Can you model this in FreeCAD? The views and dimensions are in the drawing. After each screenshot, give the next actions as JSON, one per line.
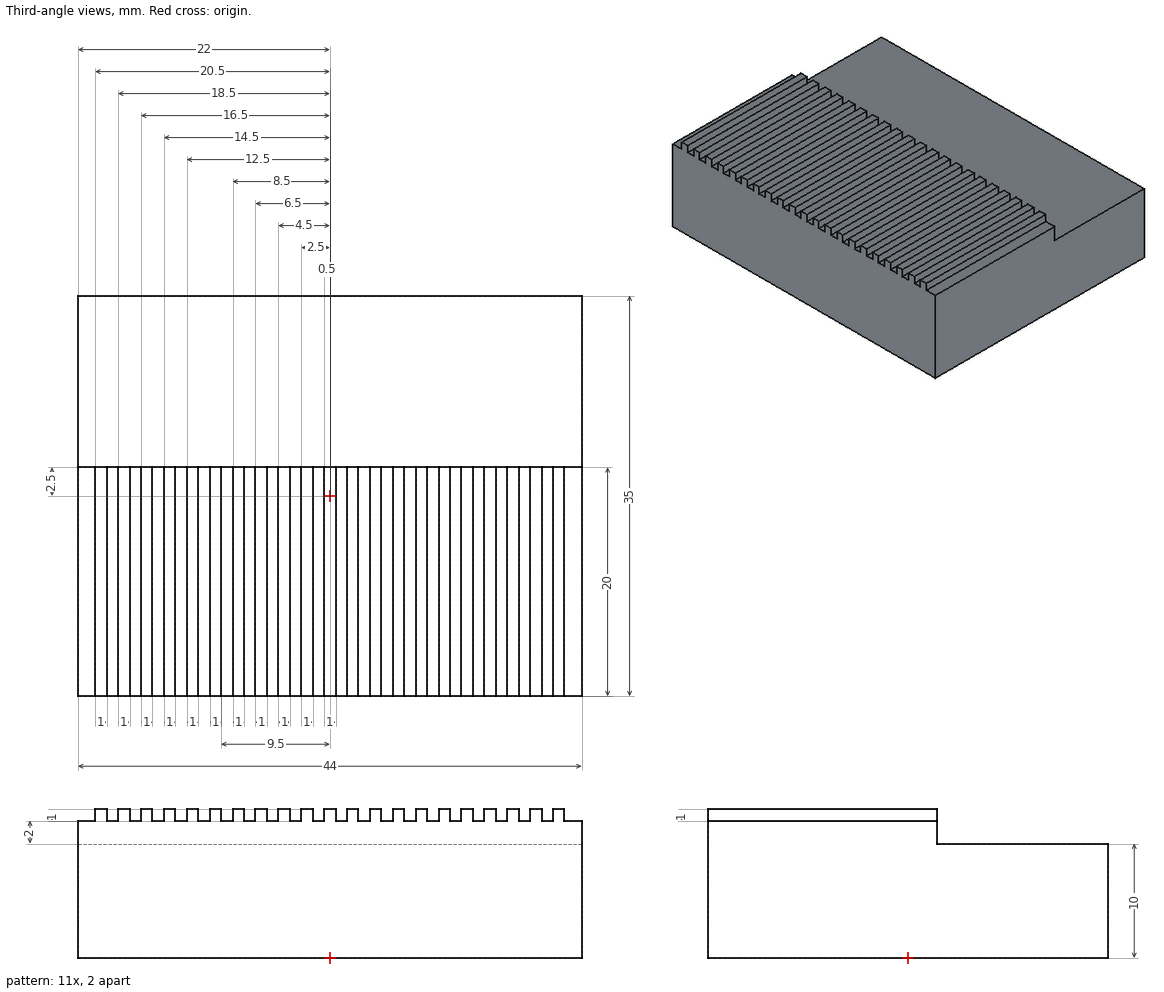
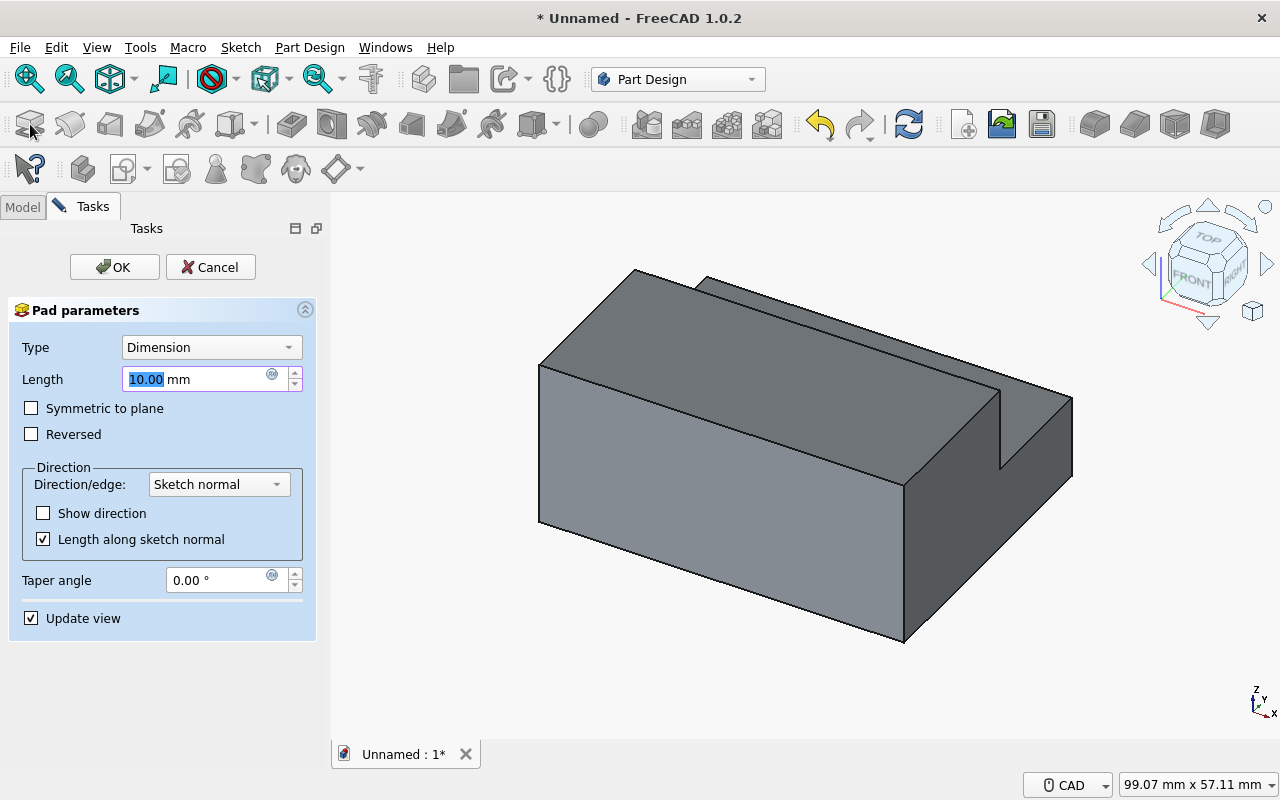
{"action": "type", "text": "2"}
{"action": "key", "text": "Tab"}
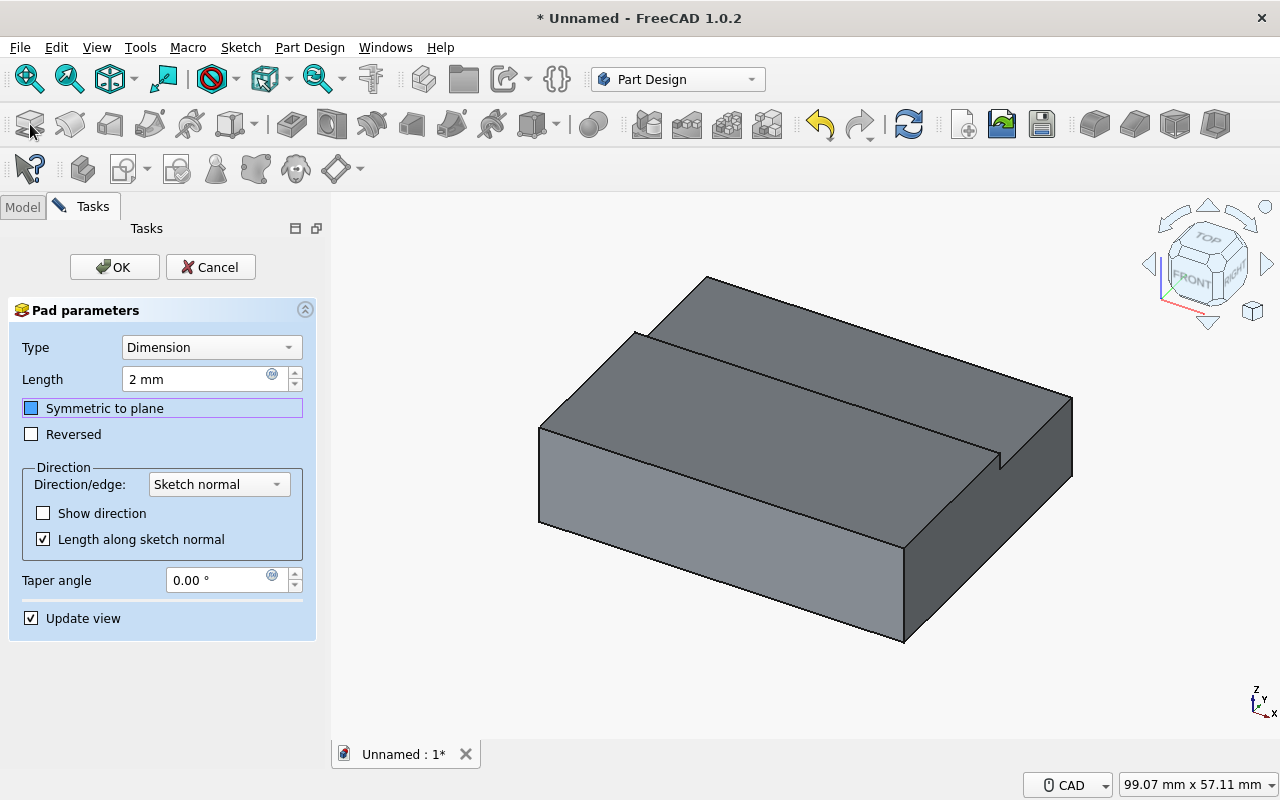
{"action": "left_click", "coordinate": [115, 267]}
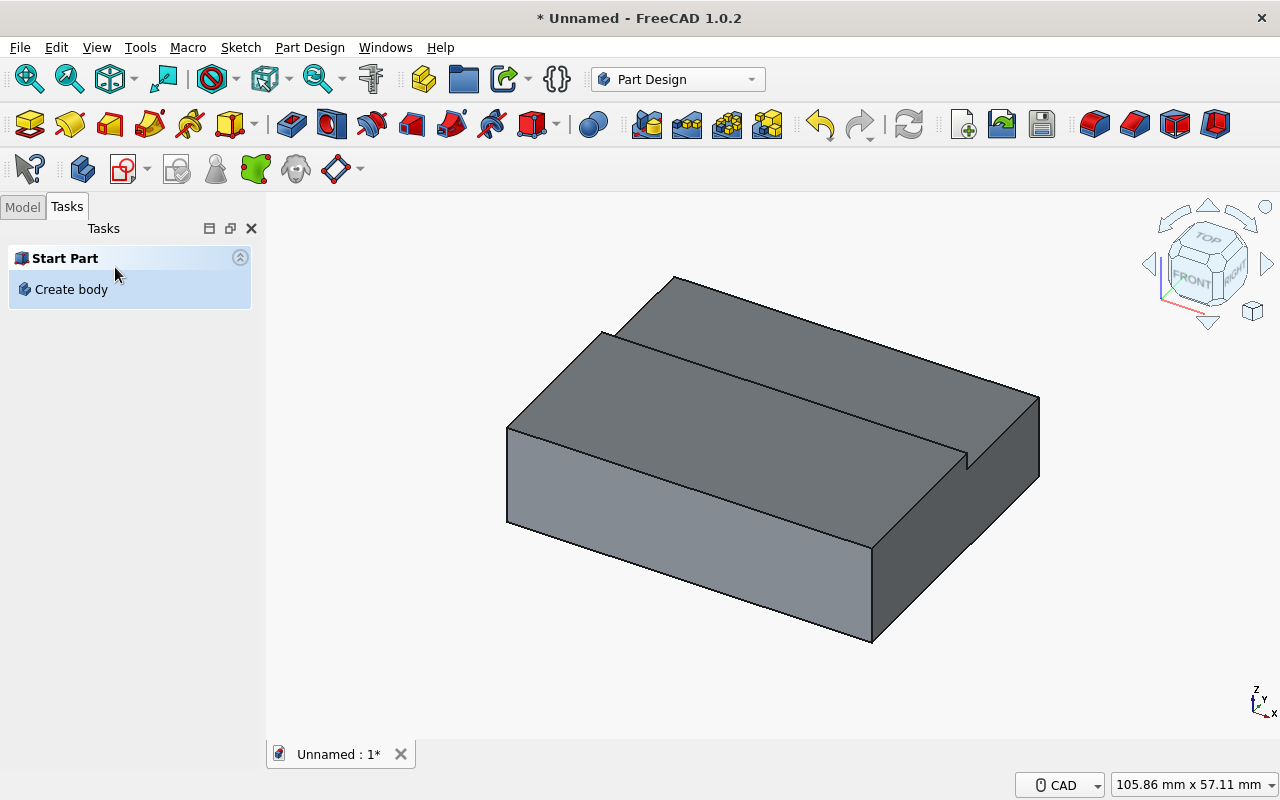
{"action": "left_click", "coordinate": [789, 457]}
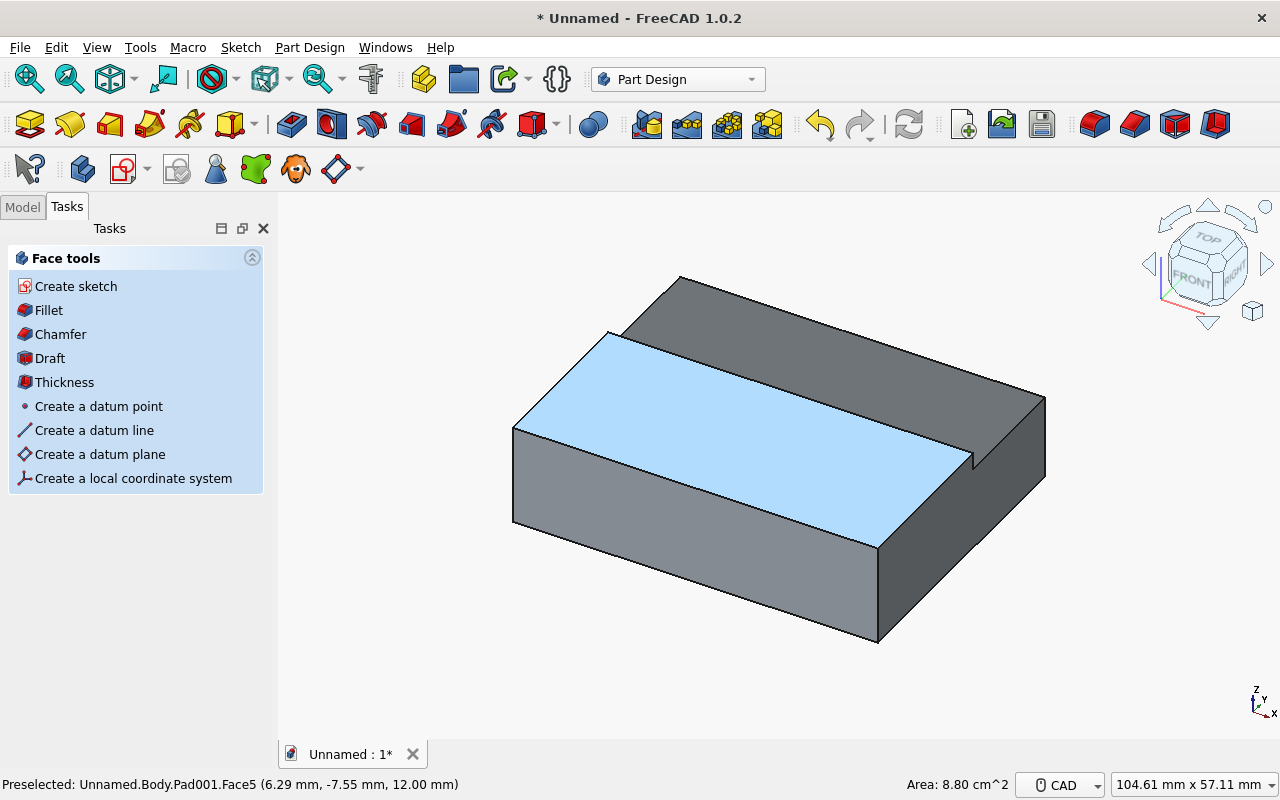
{"action": "left_click", "coordinate": [124, 170]}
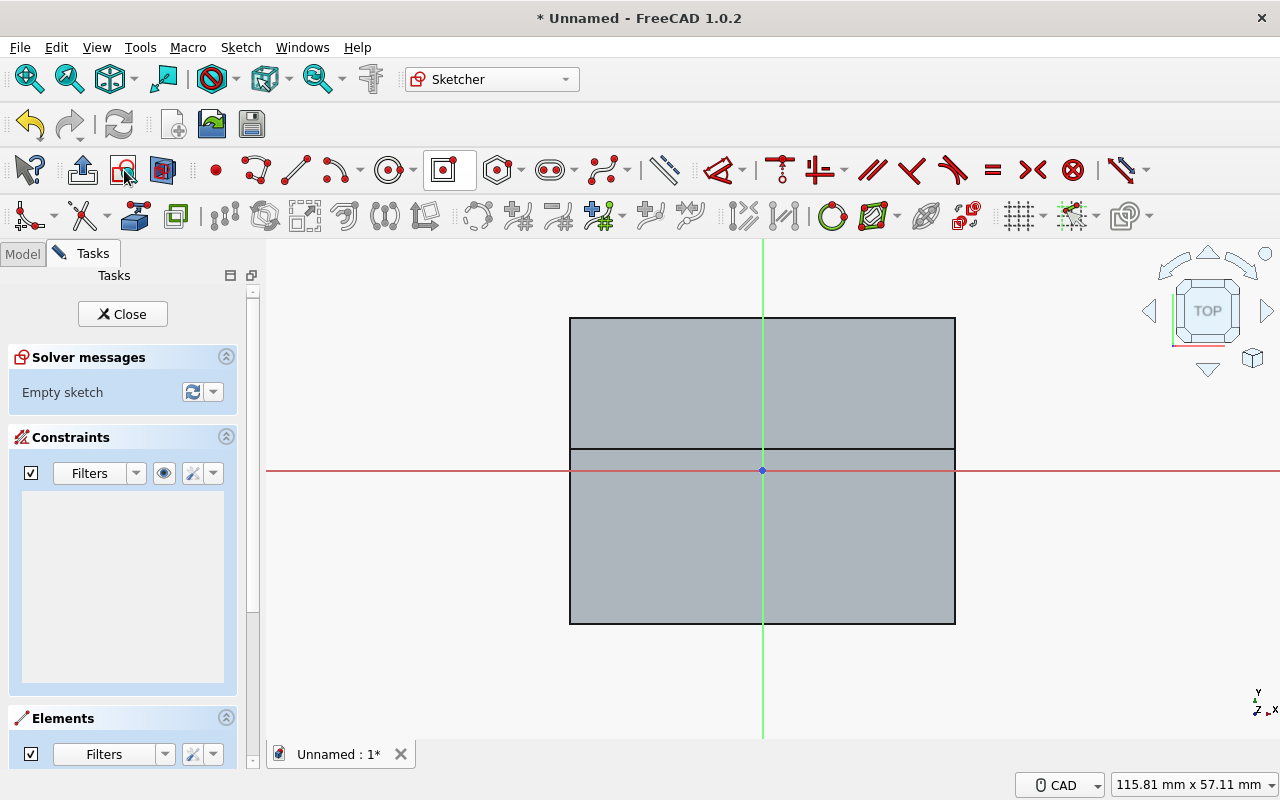
{"action": "scroll", "coordinate": [833, 594], "scroll_direction": "up", "scroll_amount": 3}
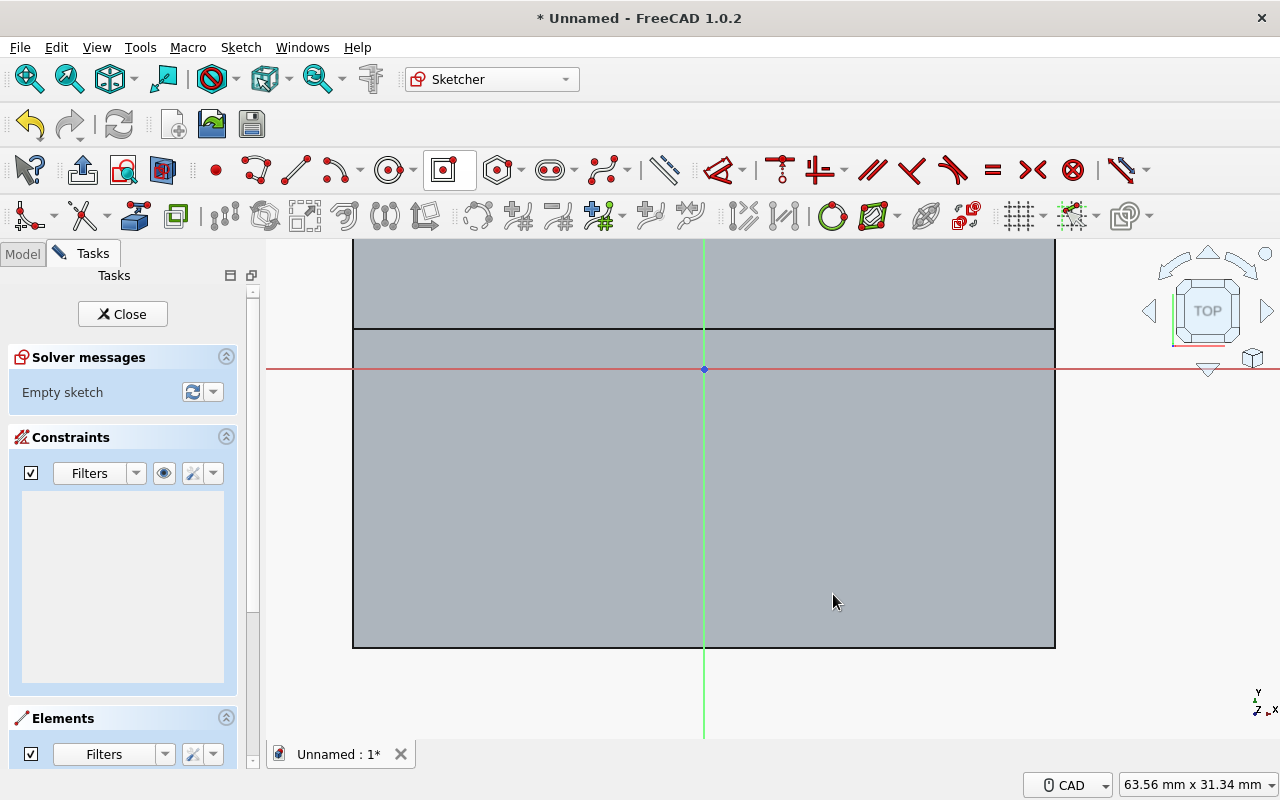
{"action": "left_click", "coordinate": [470, 170]}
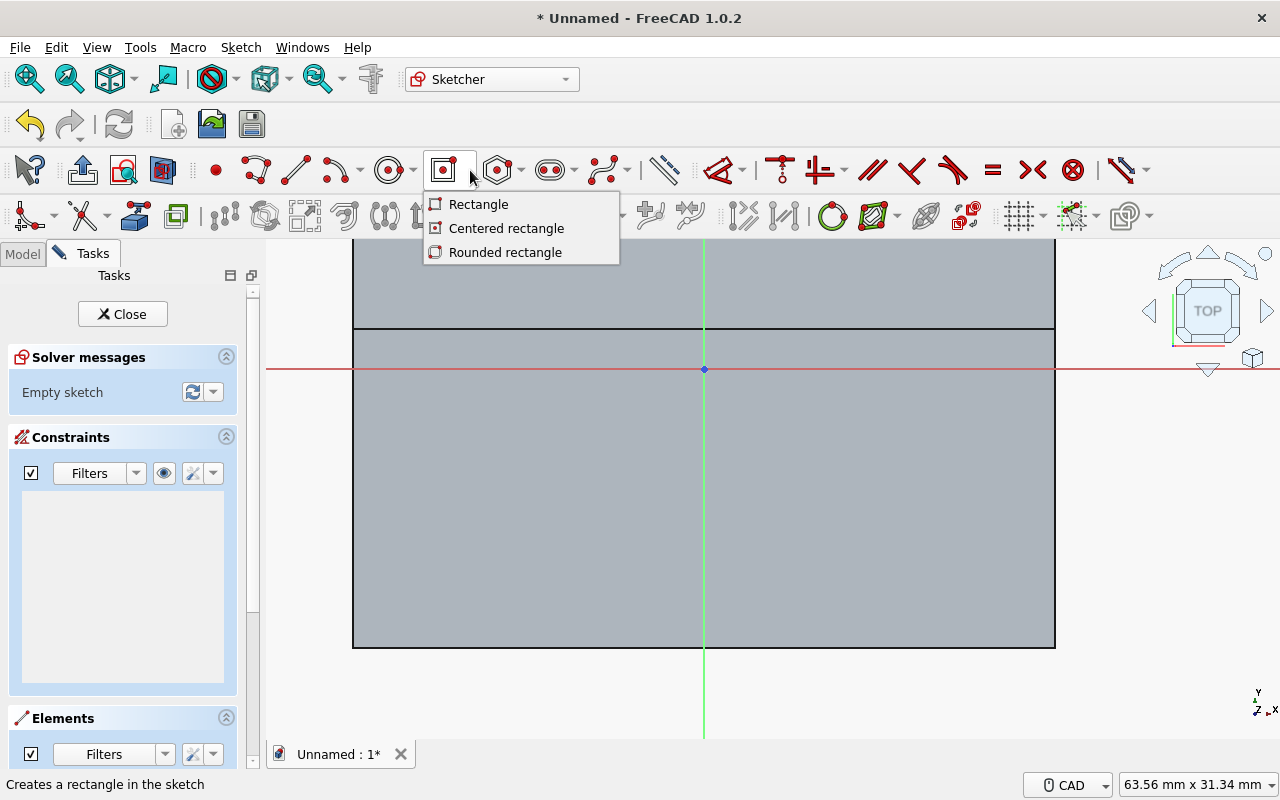
{"action": "left_click", "coordinate": [522, 204]}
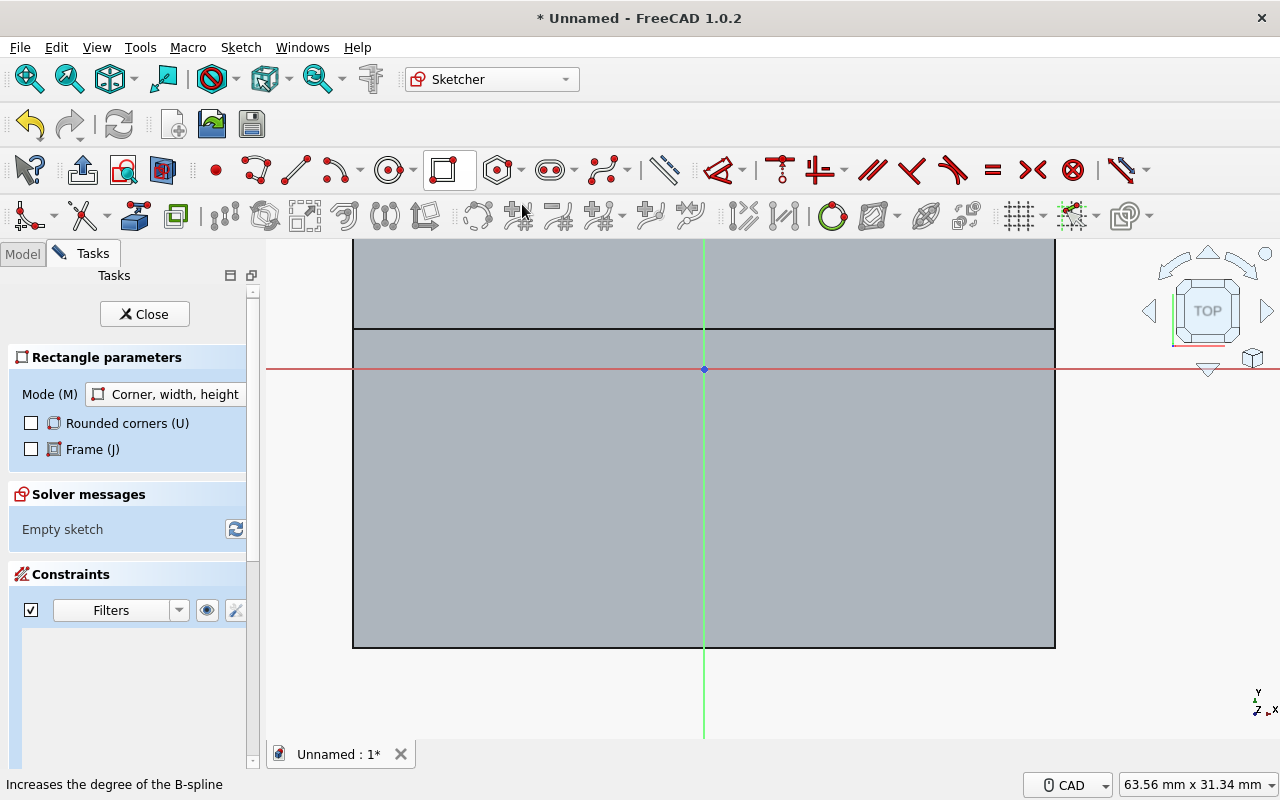
{"action": "scroll", "coordinate": [696, 329], "scroll_direction": "up", "scroll_amount": 4}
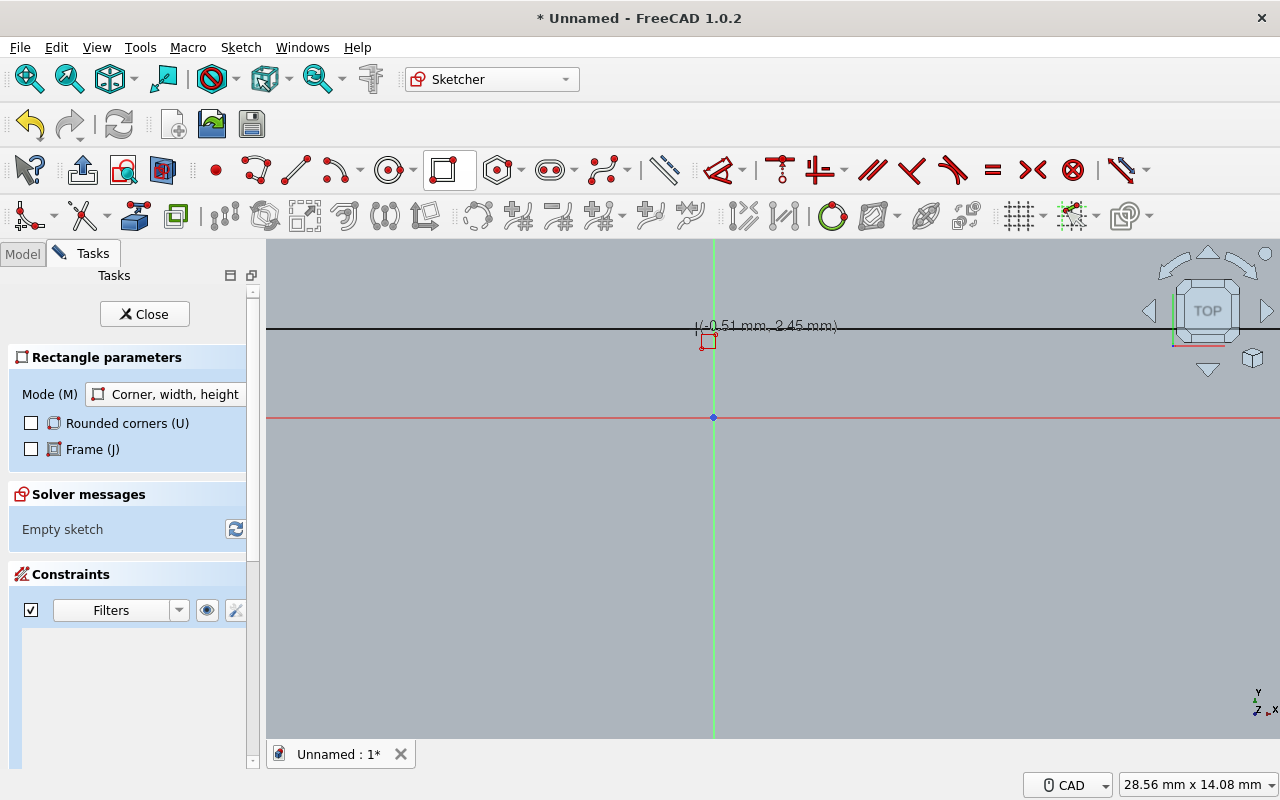
{"action": "left_click", "coordinate": [696, 329]}